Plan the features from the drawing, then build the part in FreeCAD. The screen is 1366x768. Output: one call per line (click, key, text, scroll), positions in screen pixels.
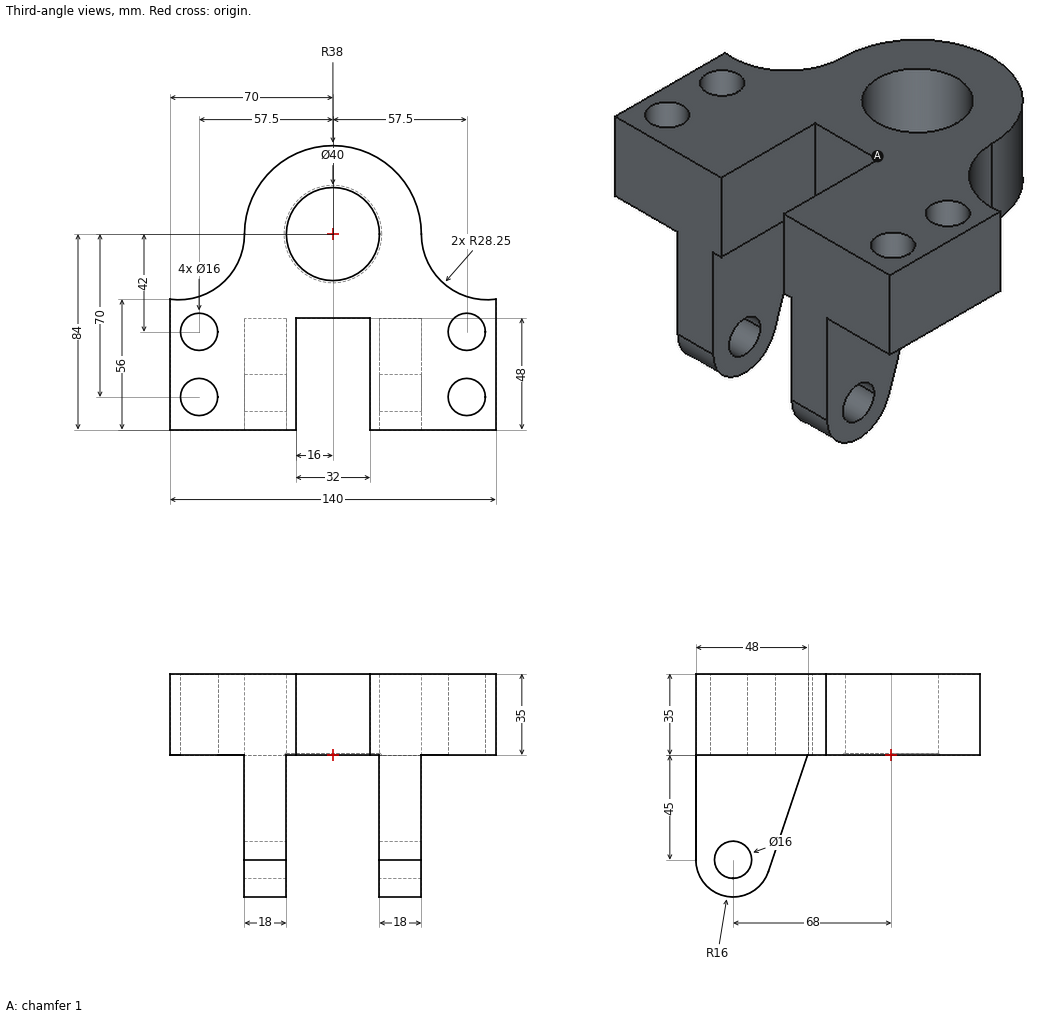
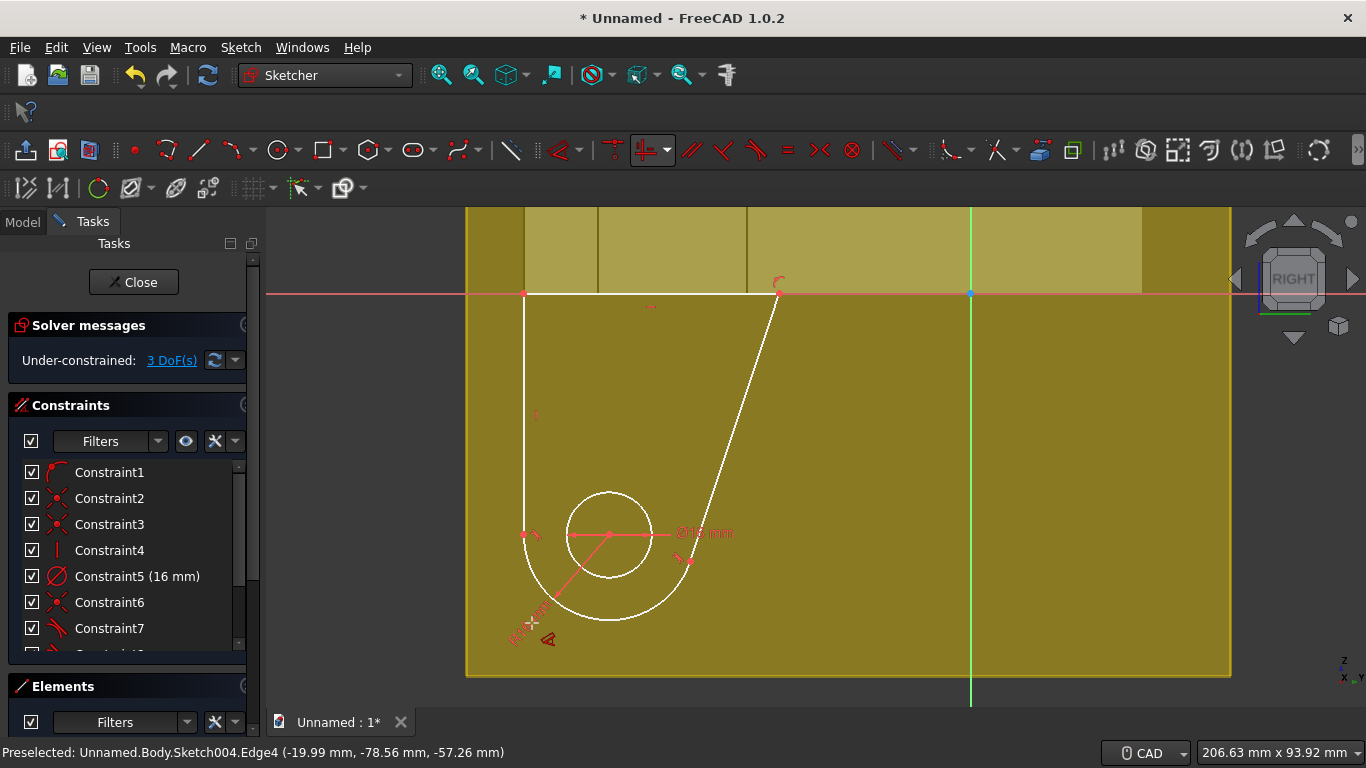
click(702, 294)
click(651, 260)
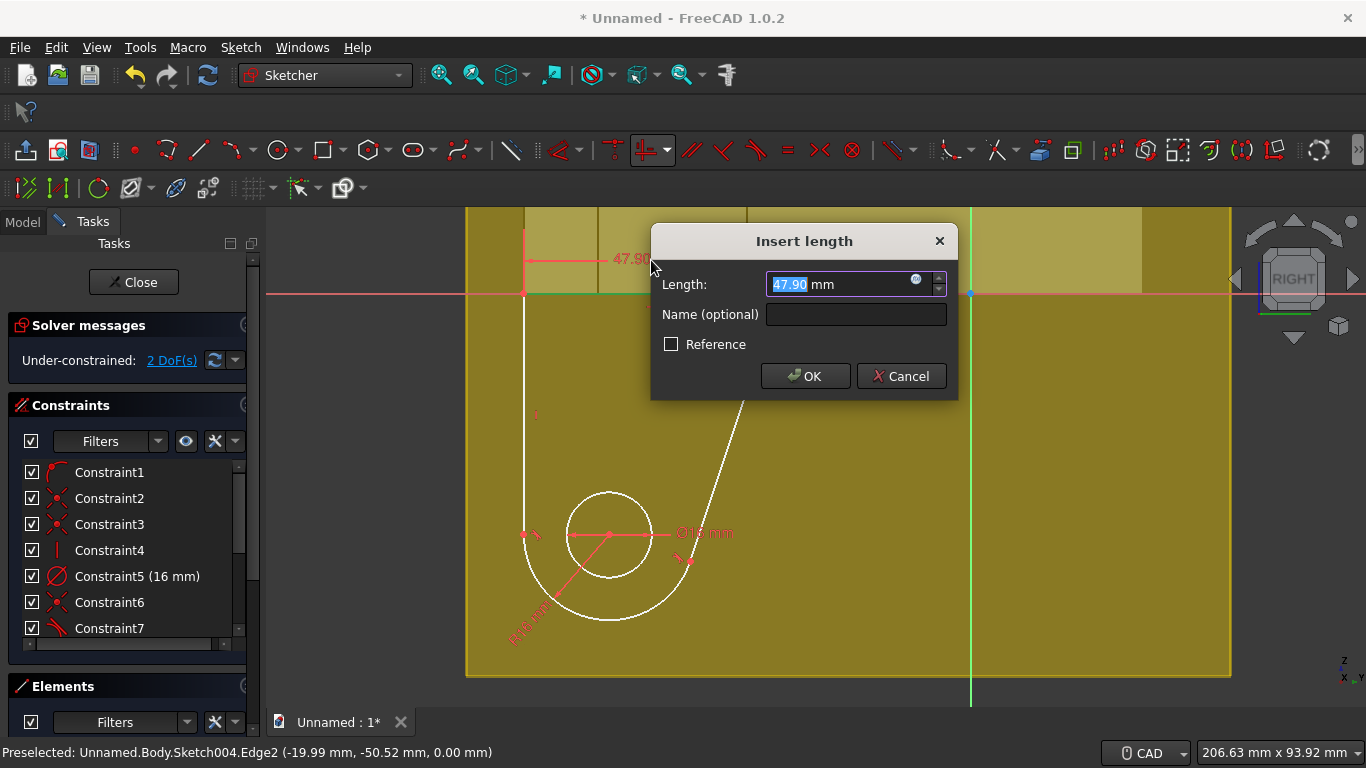
text(48)
key(Return)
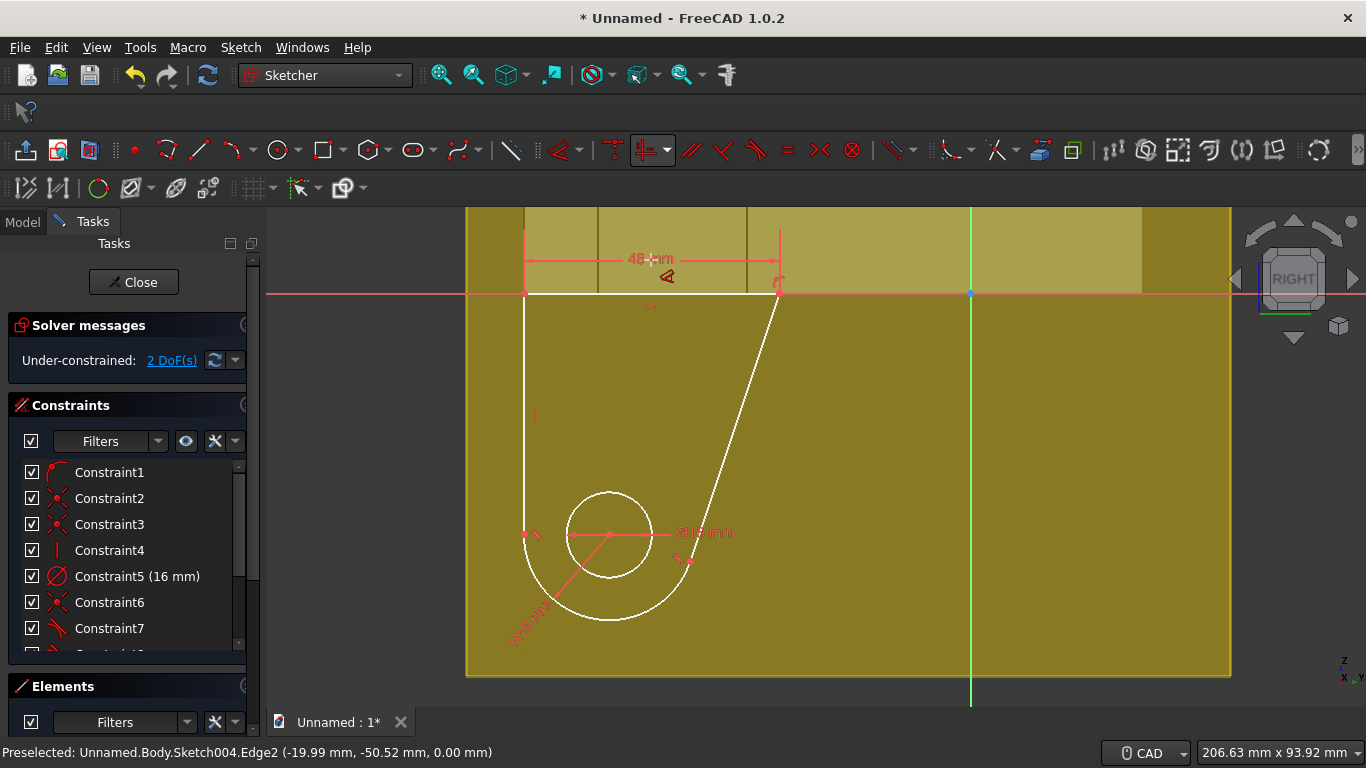
click(524, 366)
click(490, 414)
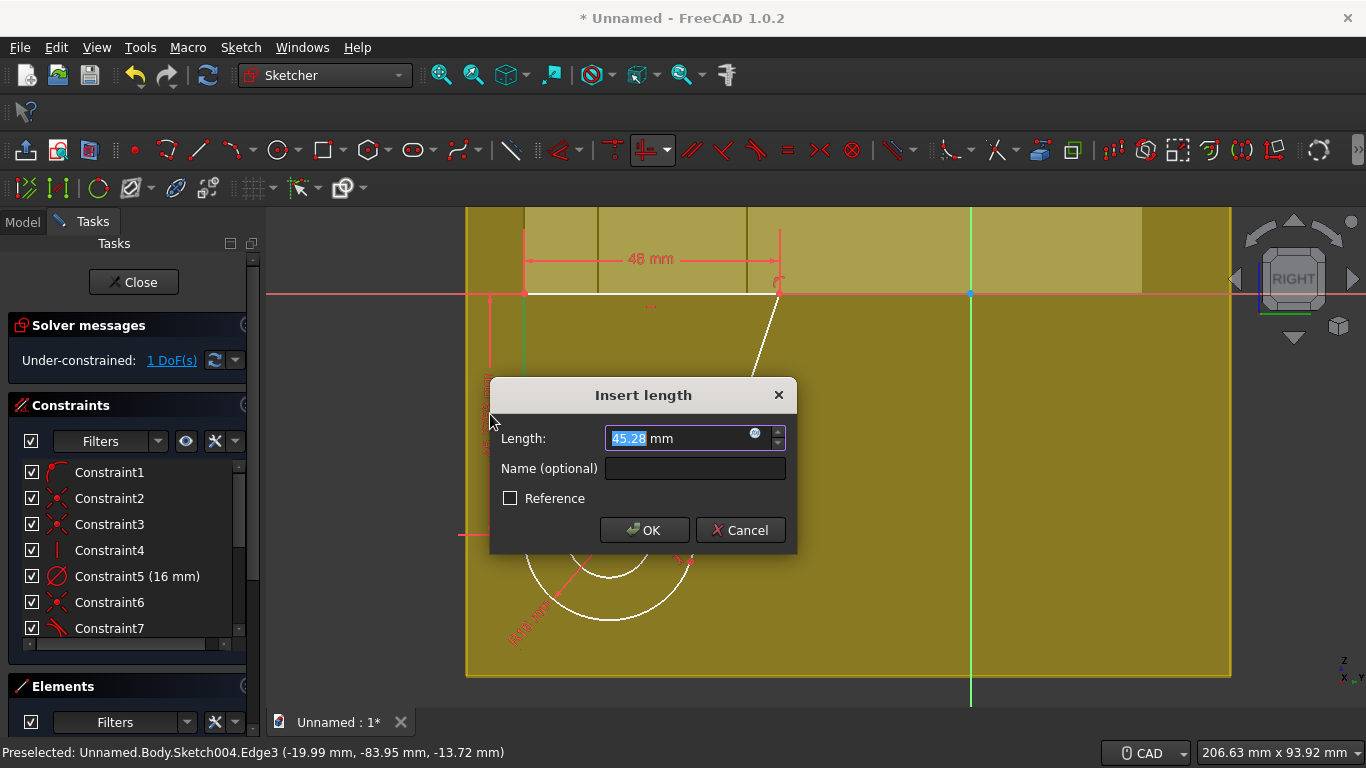
text(45)
key(Return)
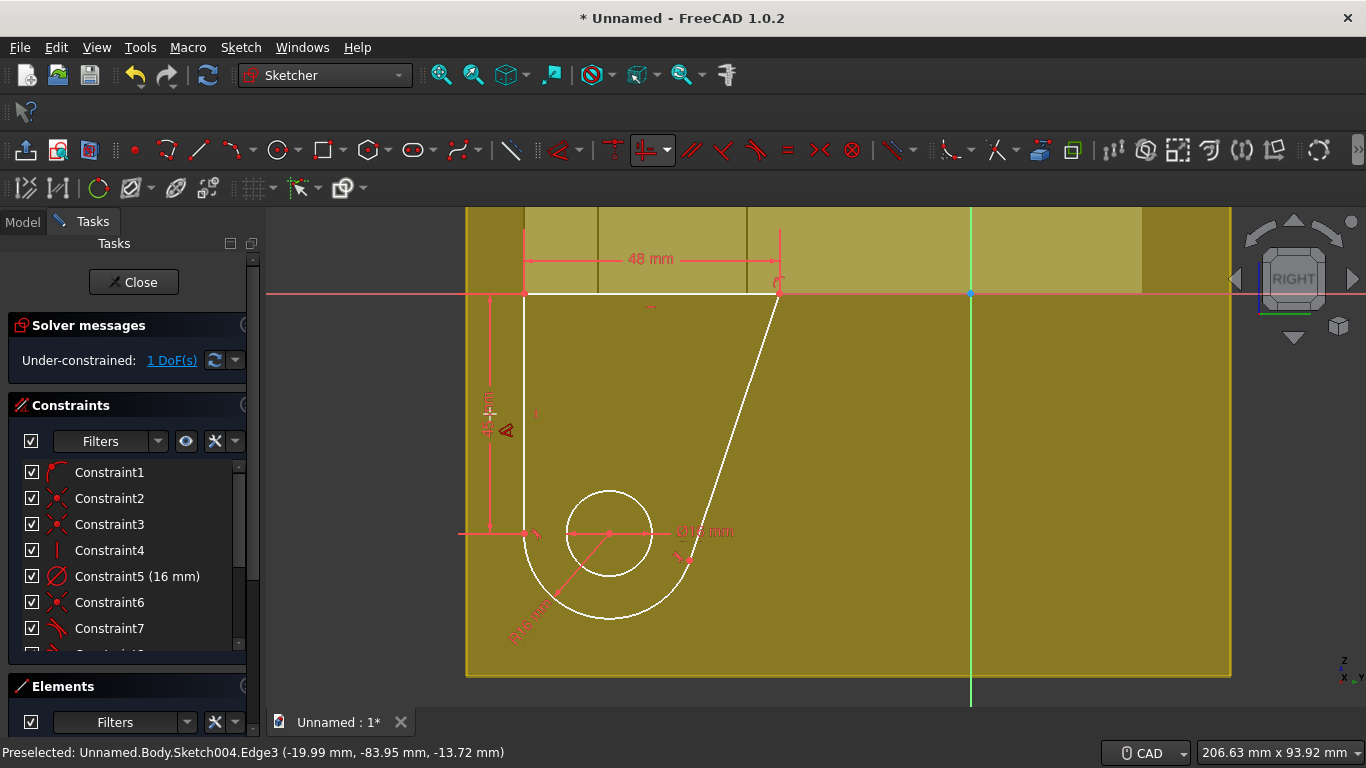
click(609, 534)
click(790, 260)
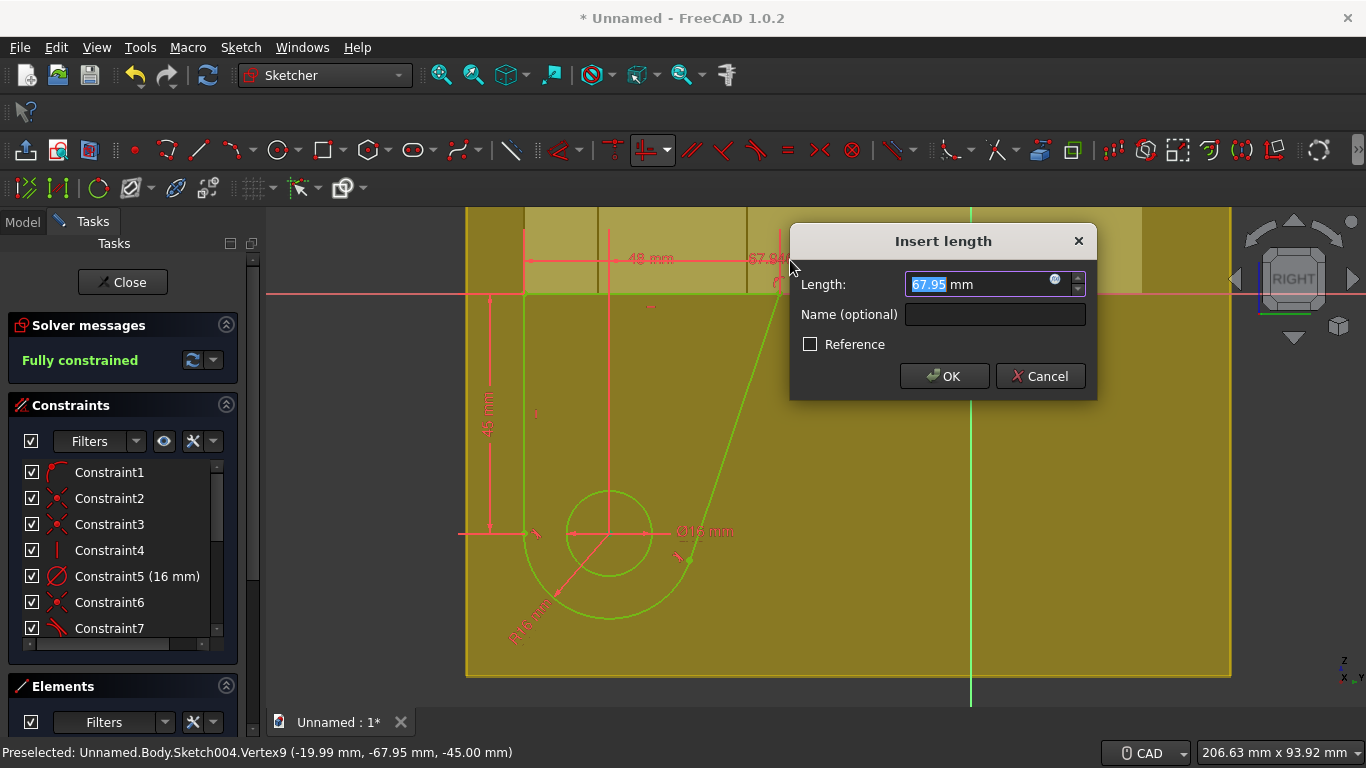
text(68)
key(Return)
key(Escape)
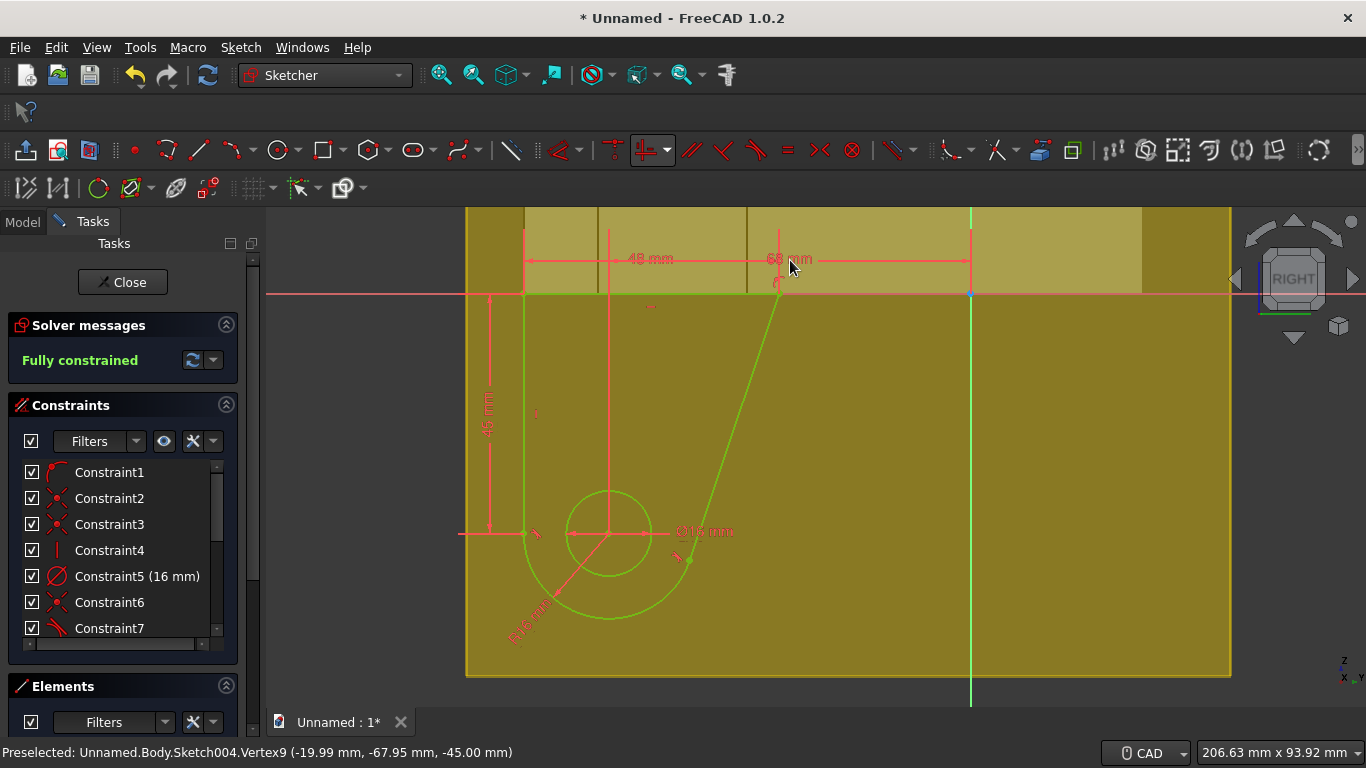
click(123, 282)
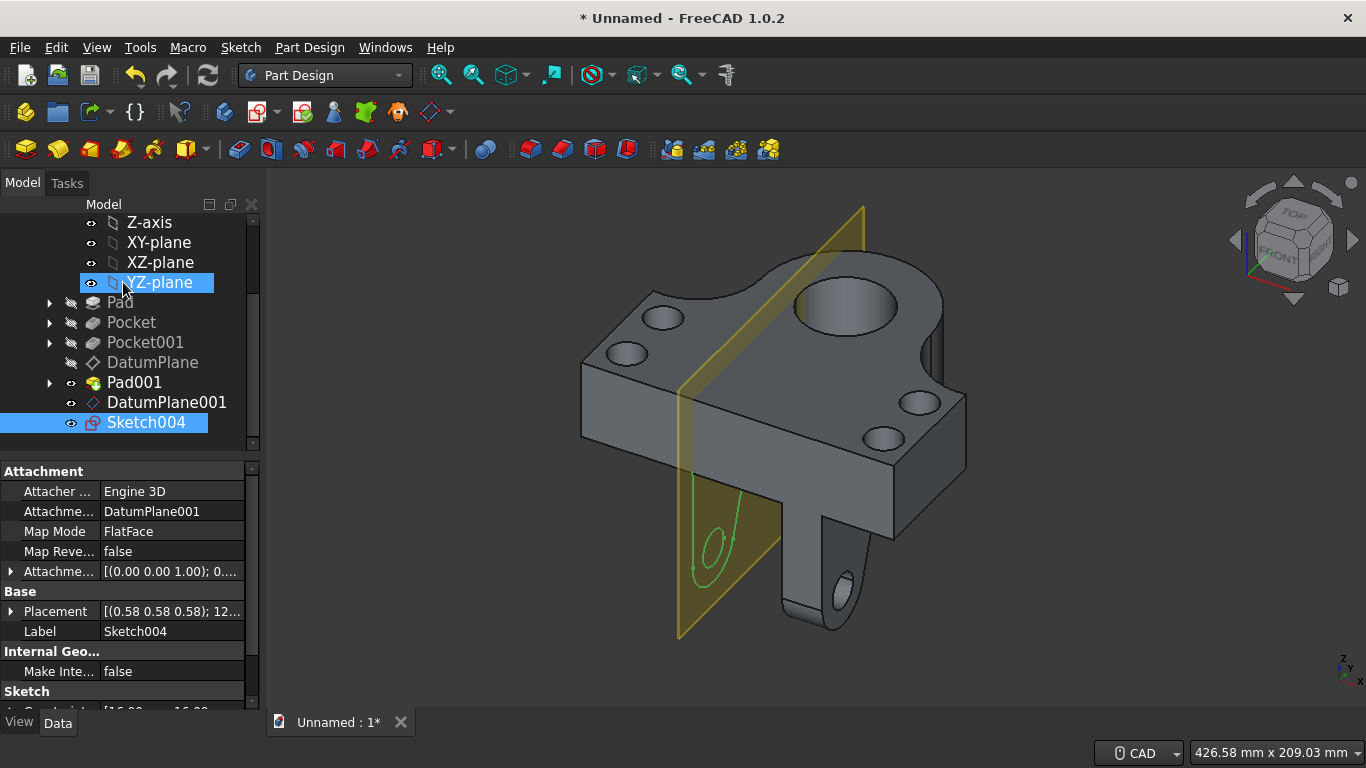
click(26, 150)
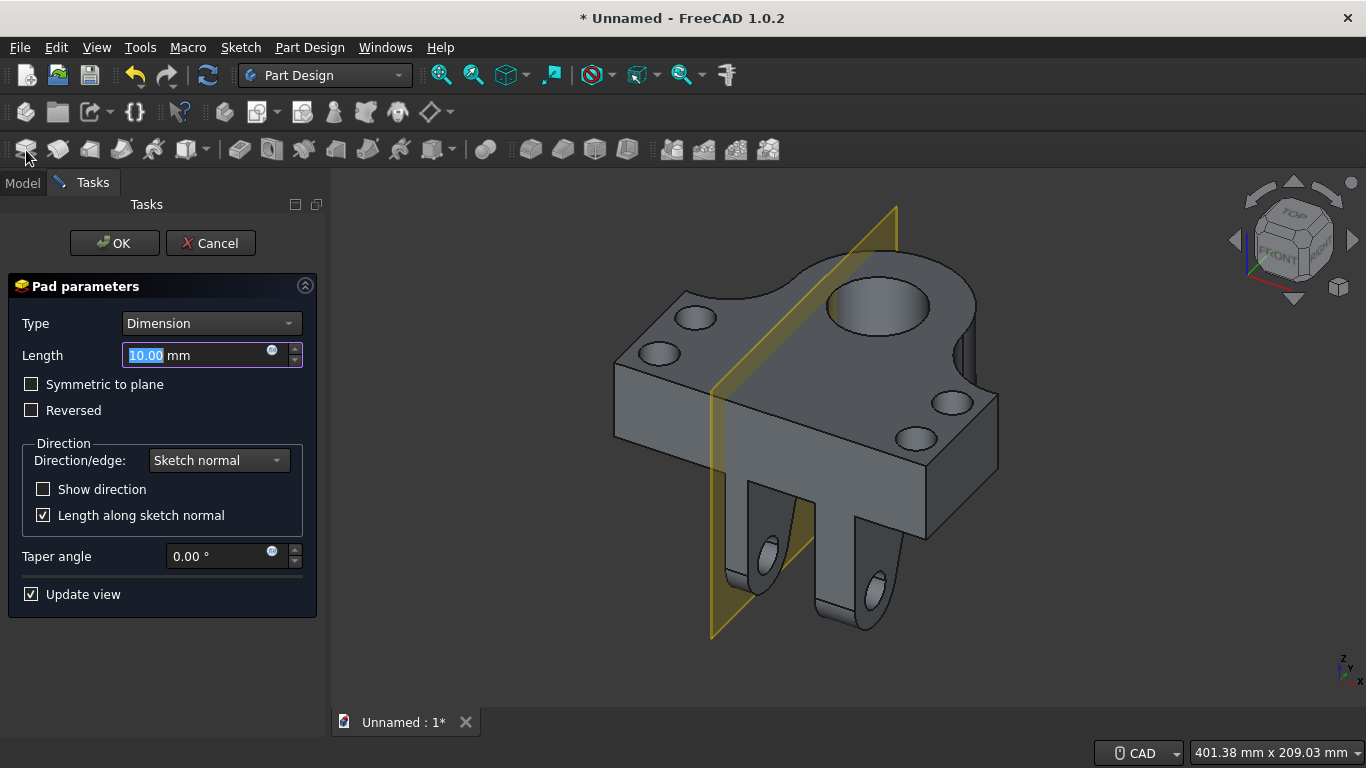
text(18)
key(Tab)